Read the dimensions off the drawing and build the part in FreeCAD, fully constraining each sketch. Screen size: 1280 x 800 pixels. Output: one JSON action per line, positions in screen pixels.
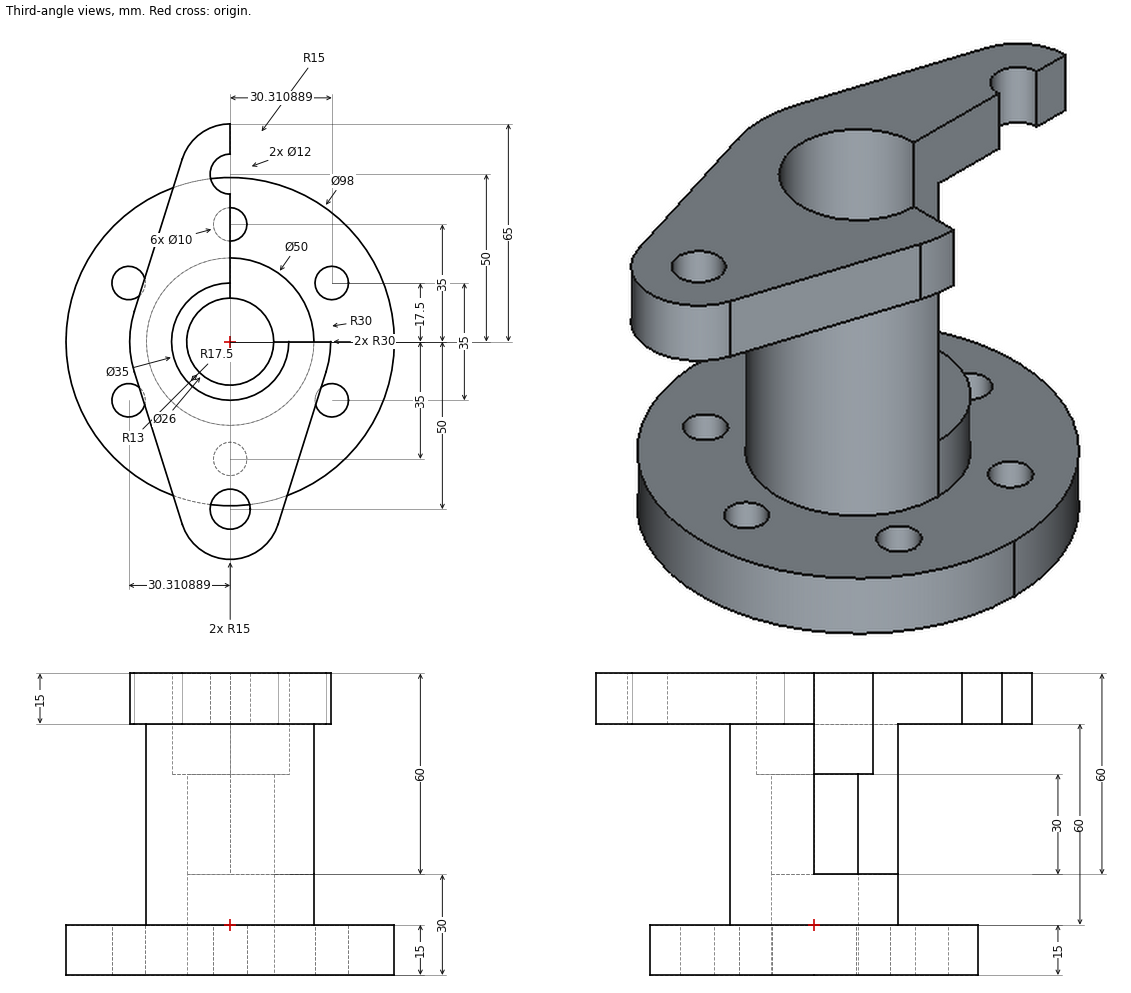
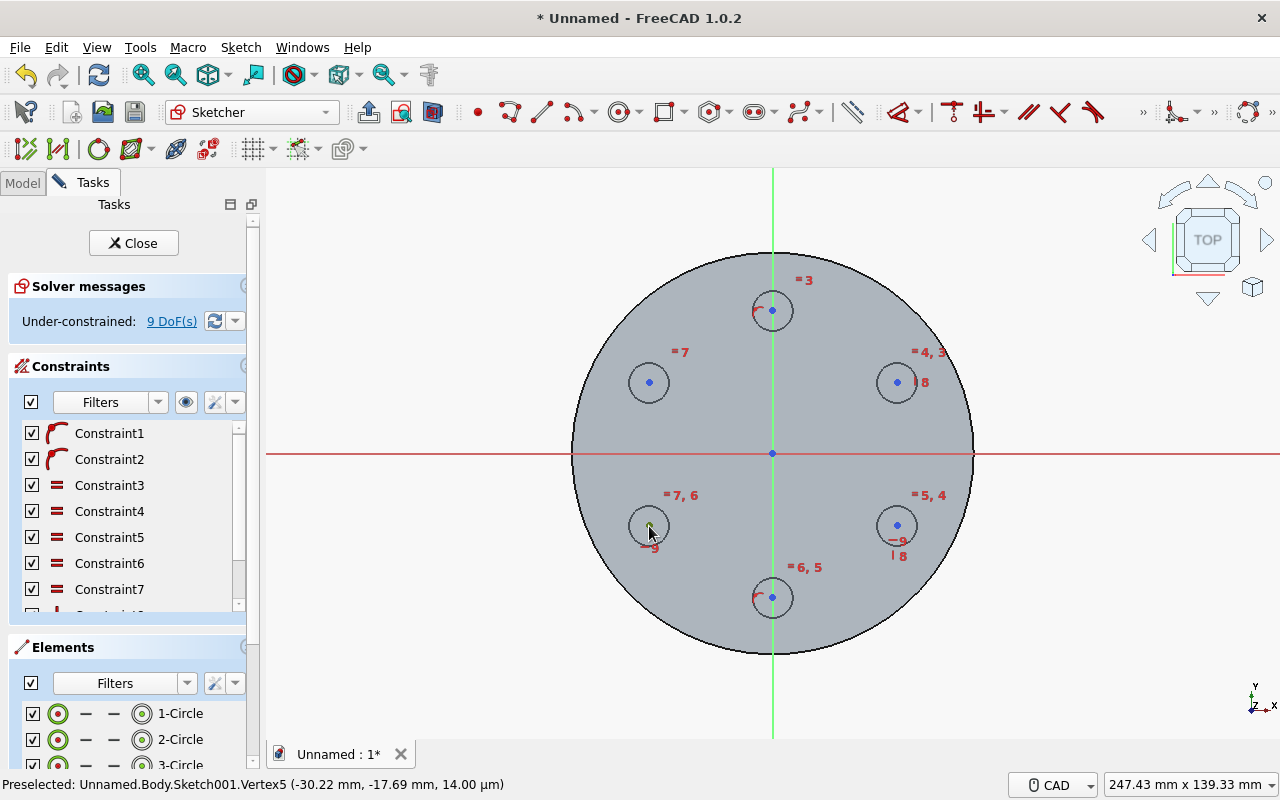
{"action": "left_click", "coordinate": [649, 383]}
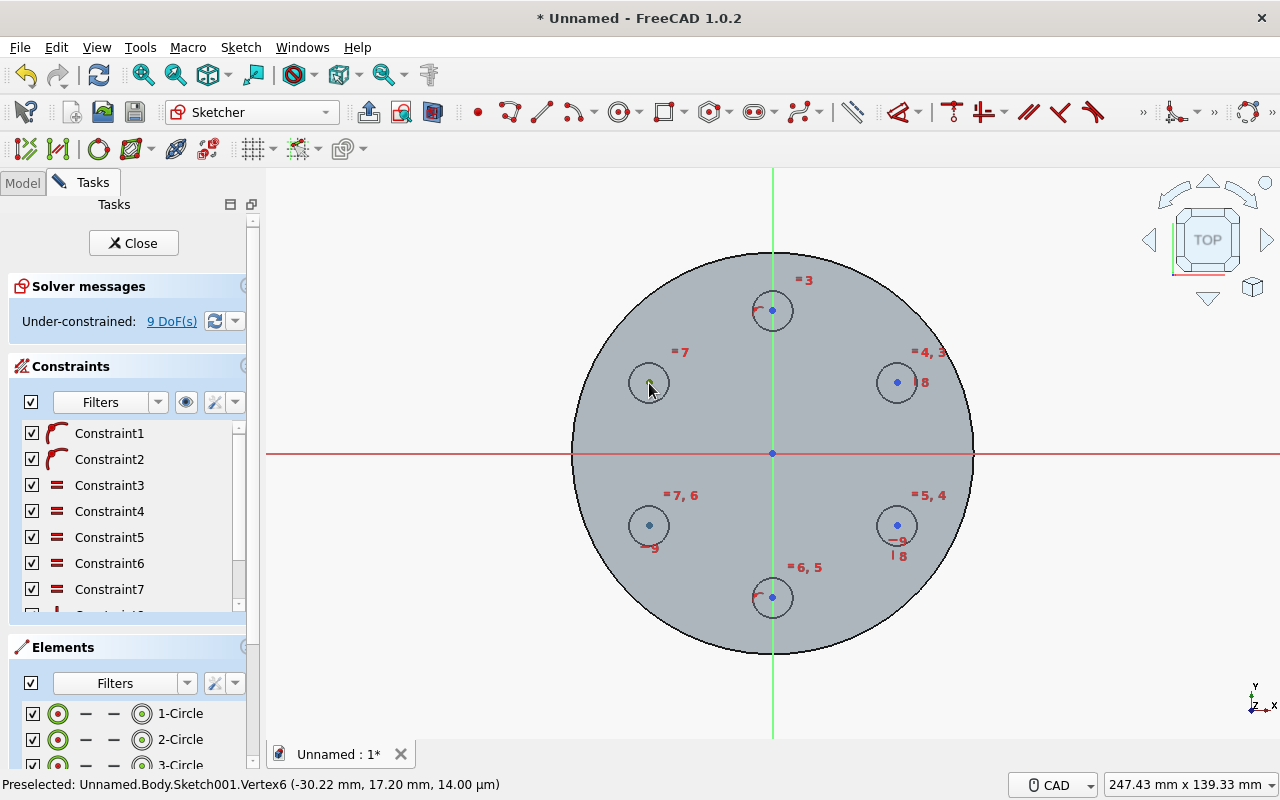
{"action": "left_click", "coordinate": [1006, 112]}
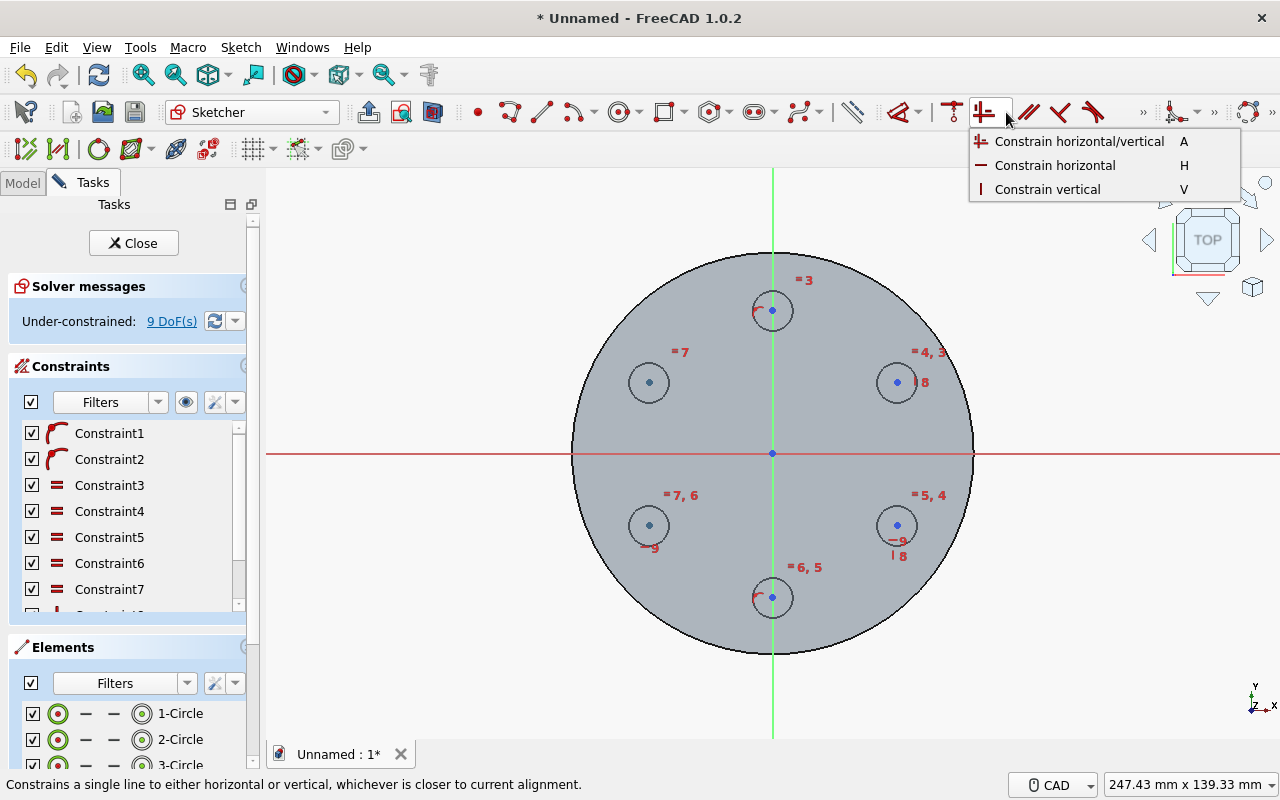
{"action": "left_click", "coordinate": [1105, 189]}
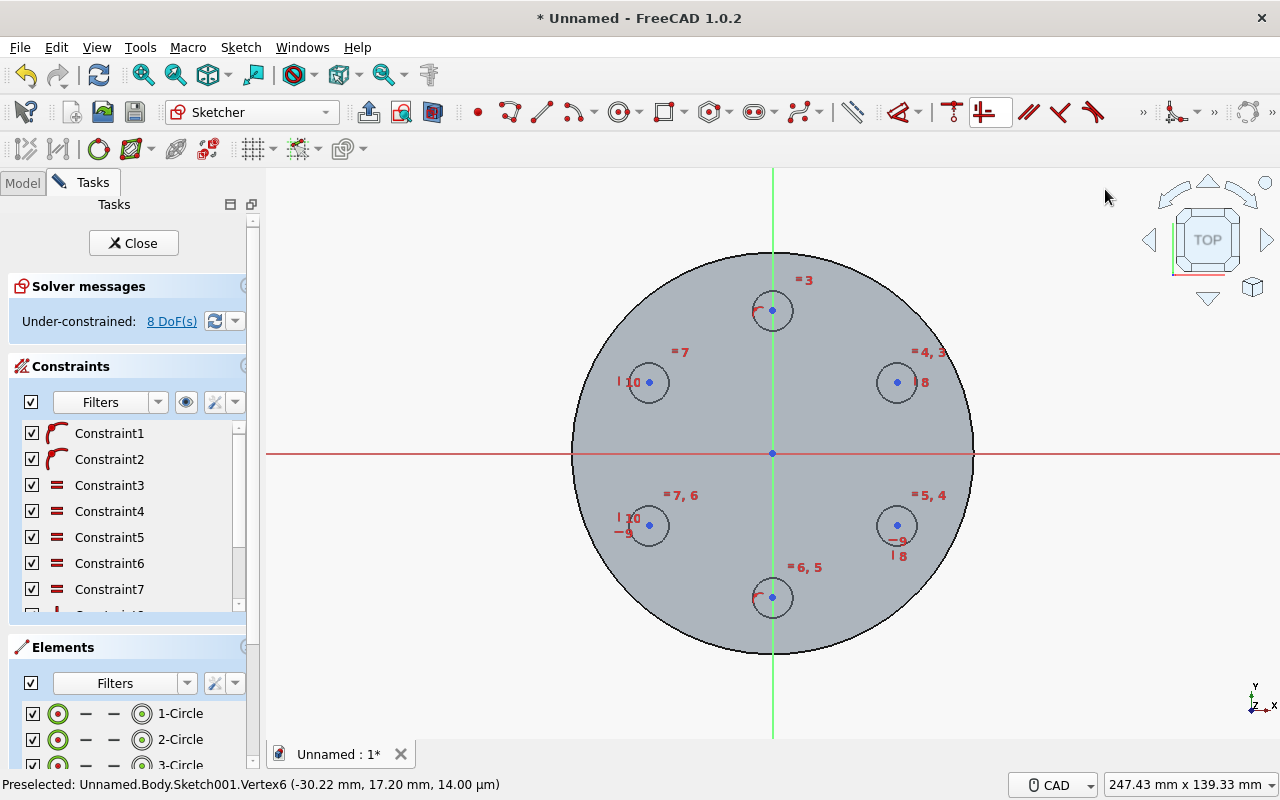
{"action": "left_click", "coordinate": [897, 383]}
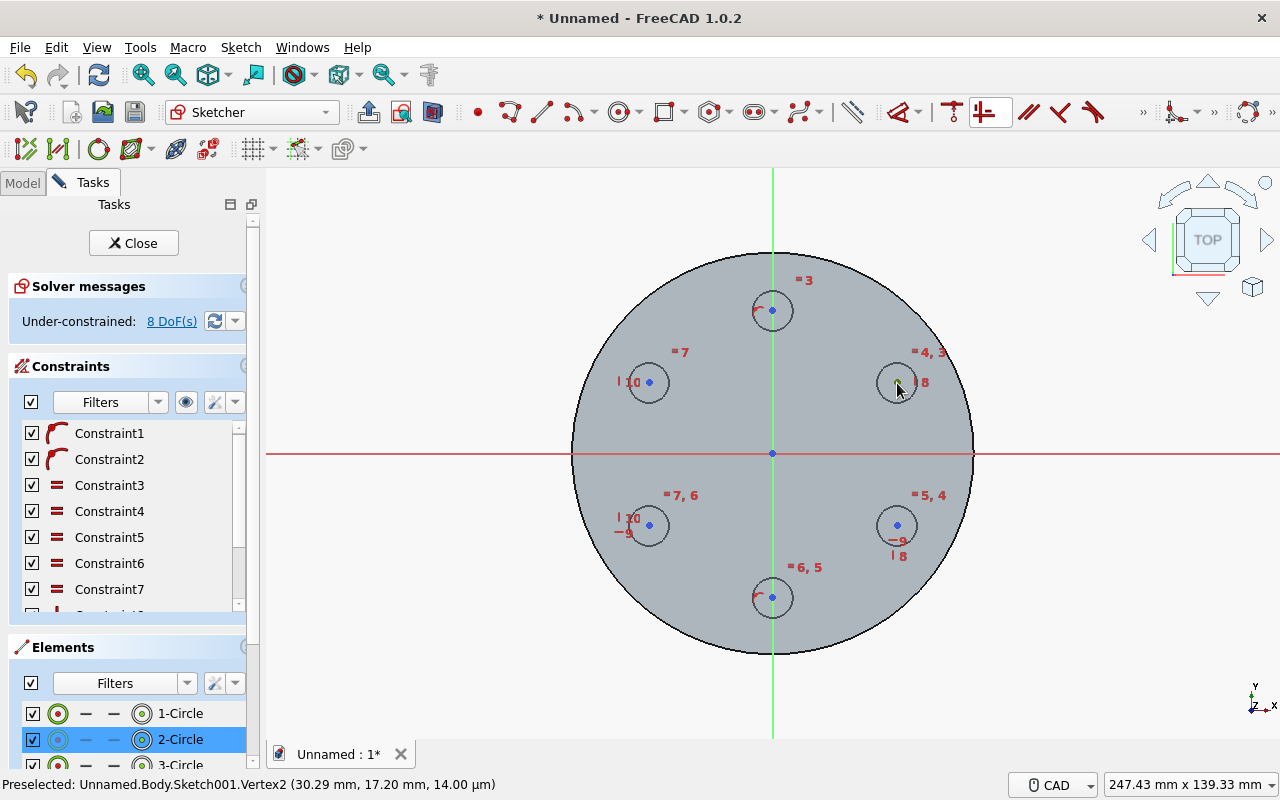
{"action": "left_click", "coordinate": [649, 383]}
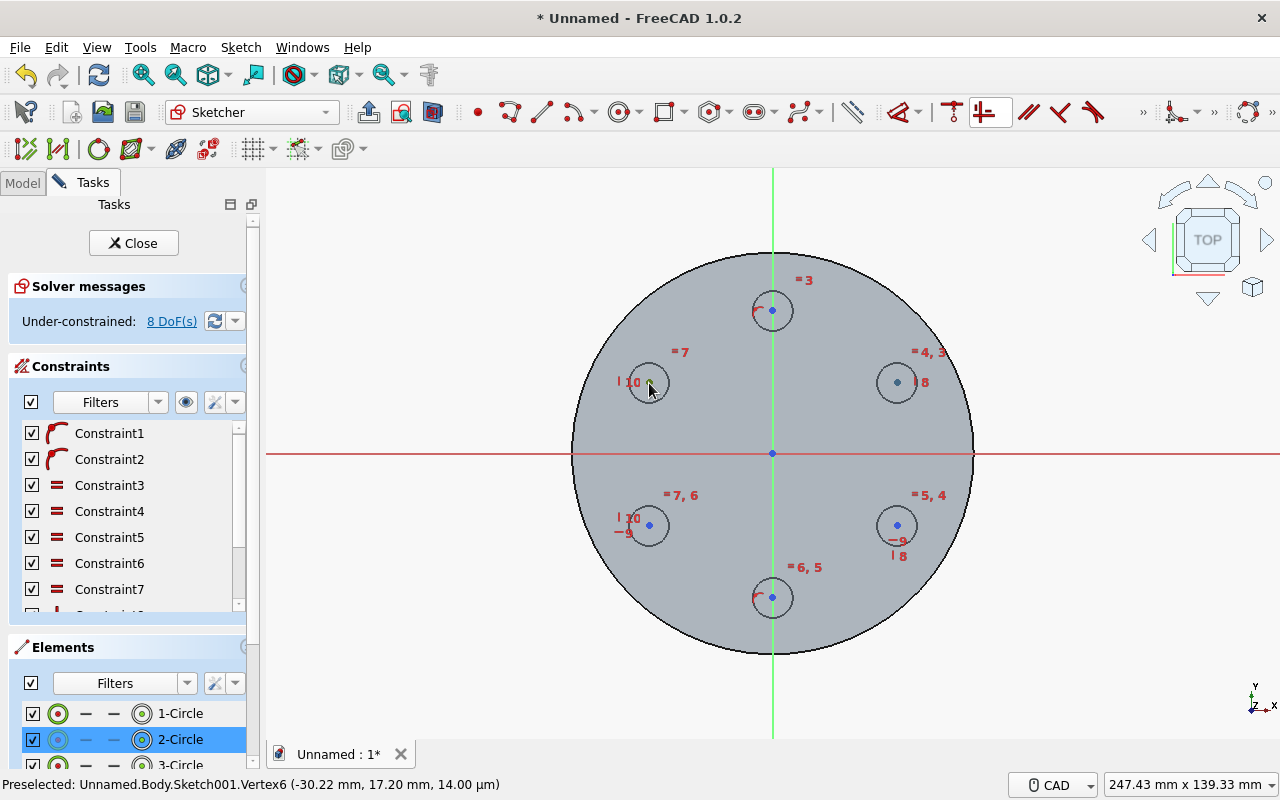
{"action": "left_click", "coordinate": [1006, 112]}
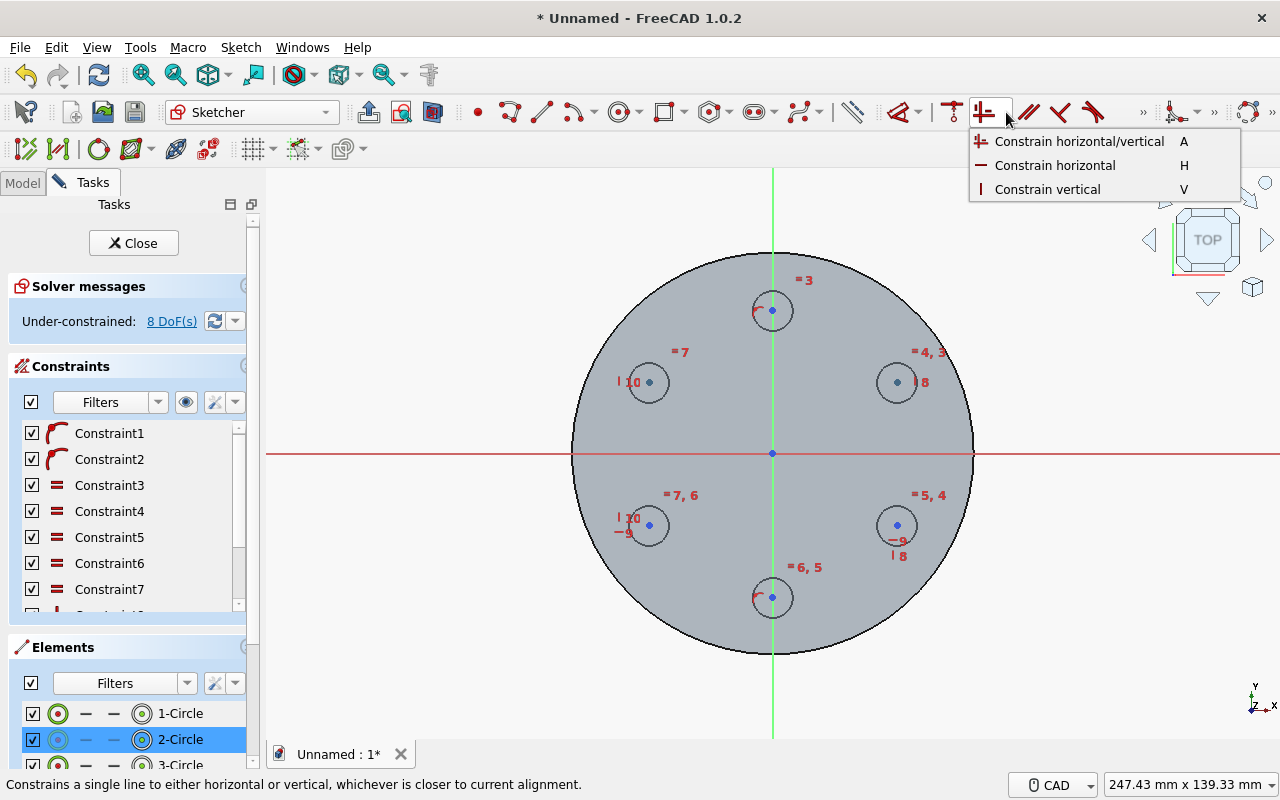
{"action": "left_click", "coordinate": [1105, 165]}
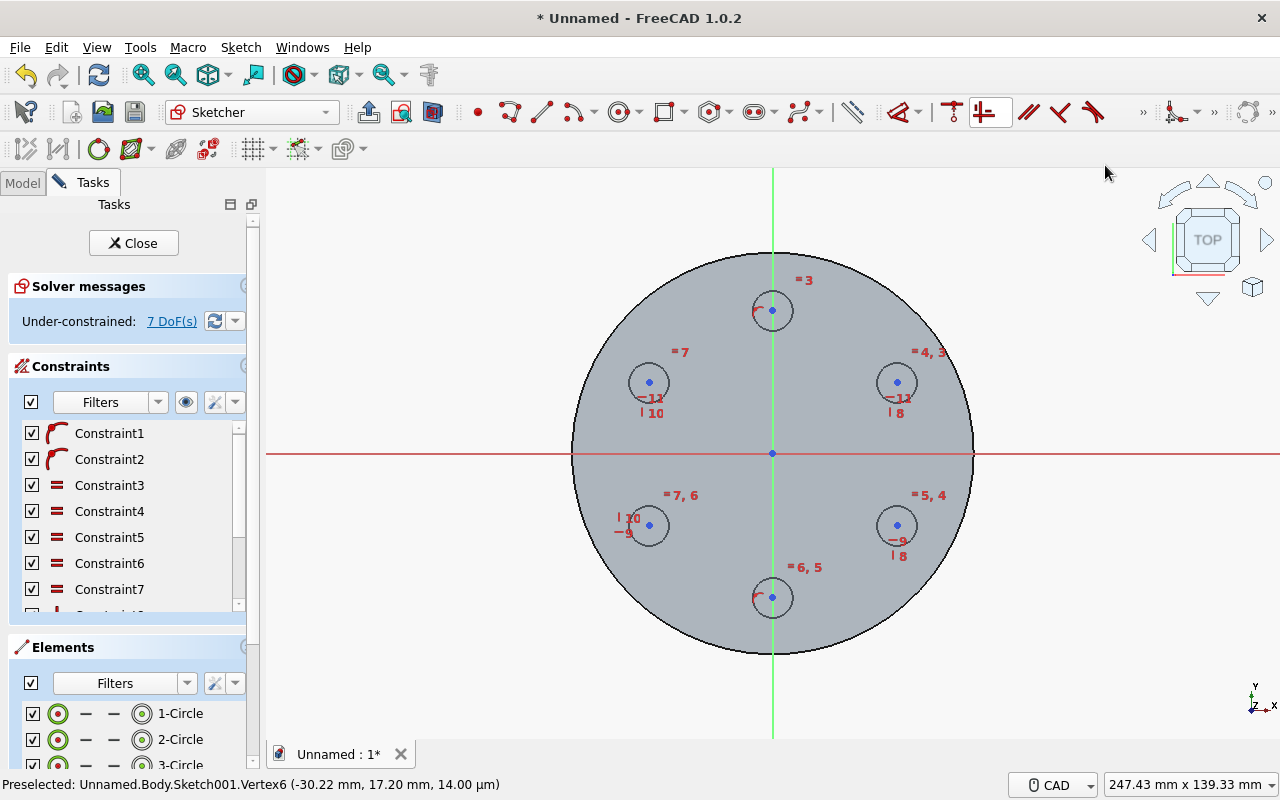
{"action": "left_click", "coordinate": [787, 297]}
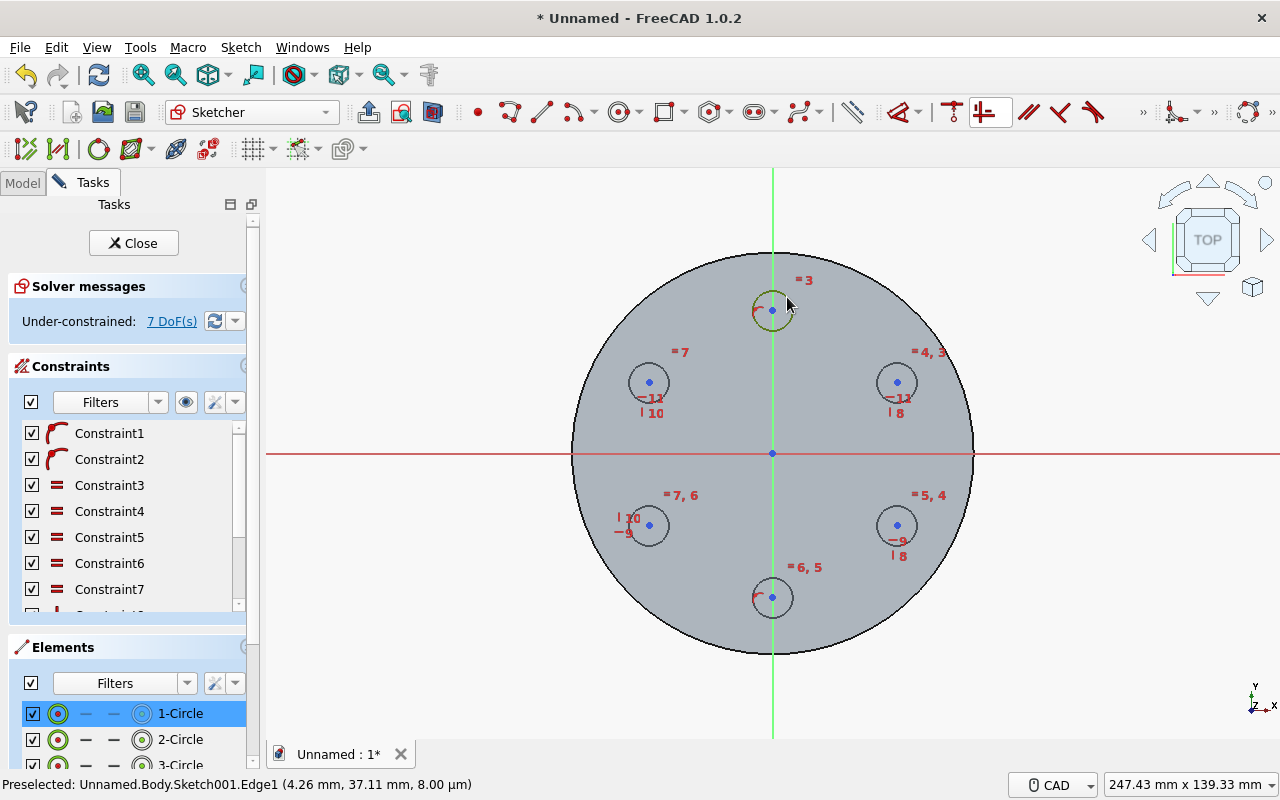
{"action": "key", "text": "k o"}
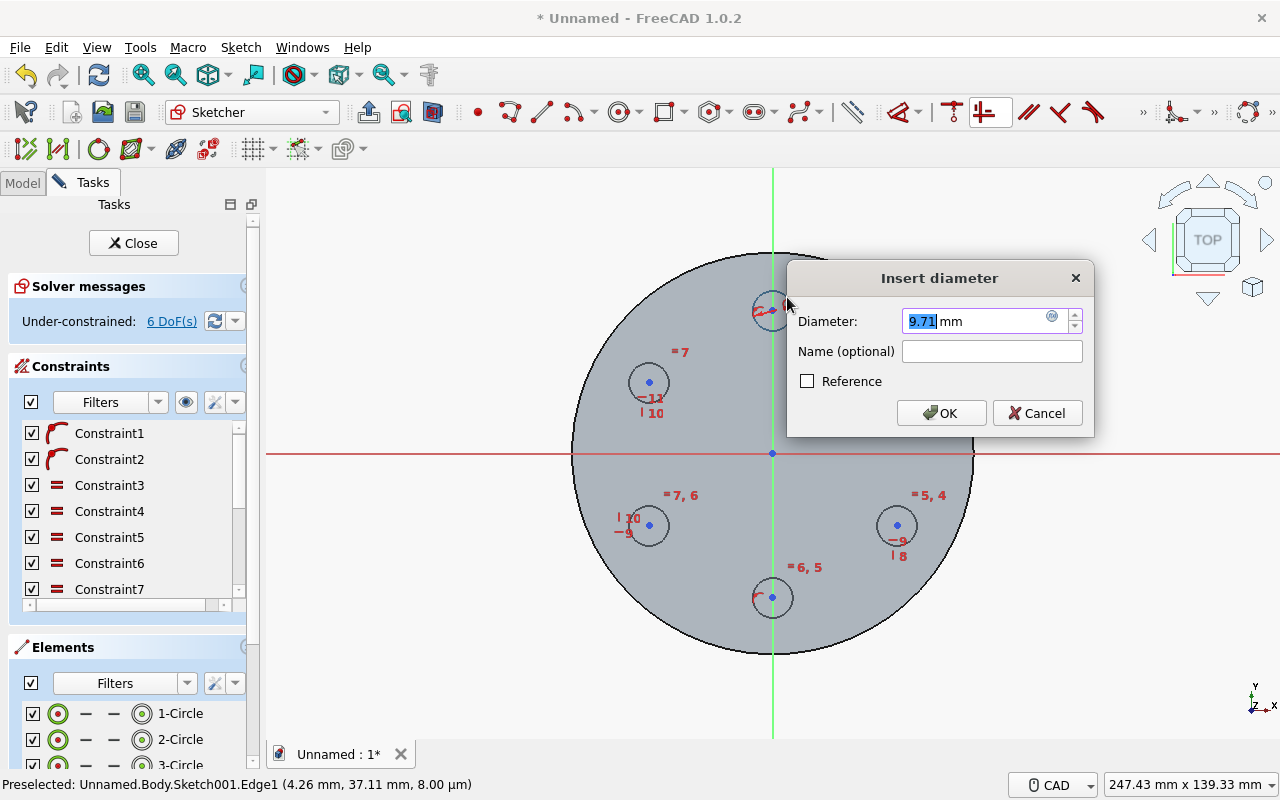
{"action": "type", "text": "10"}
{"action": "key", "text": "Return"}